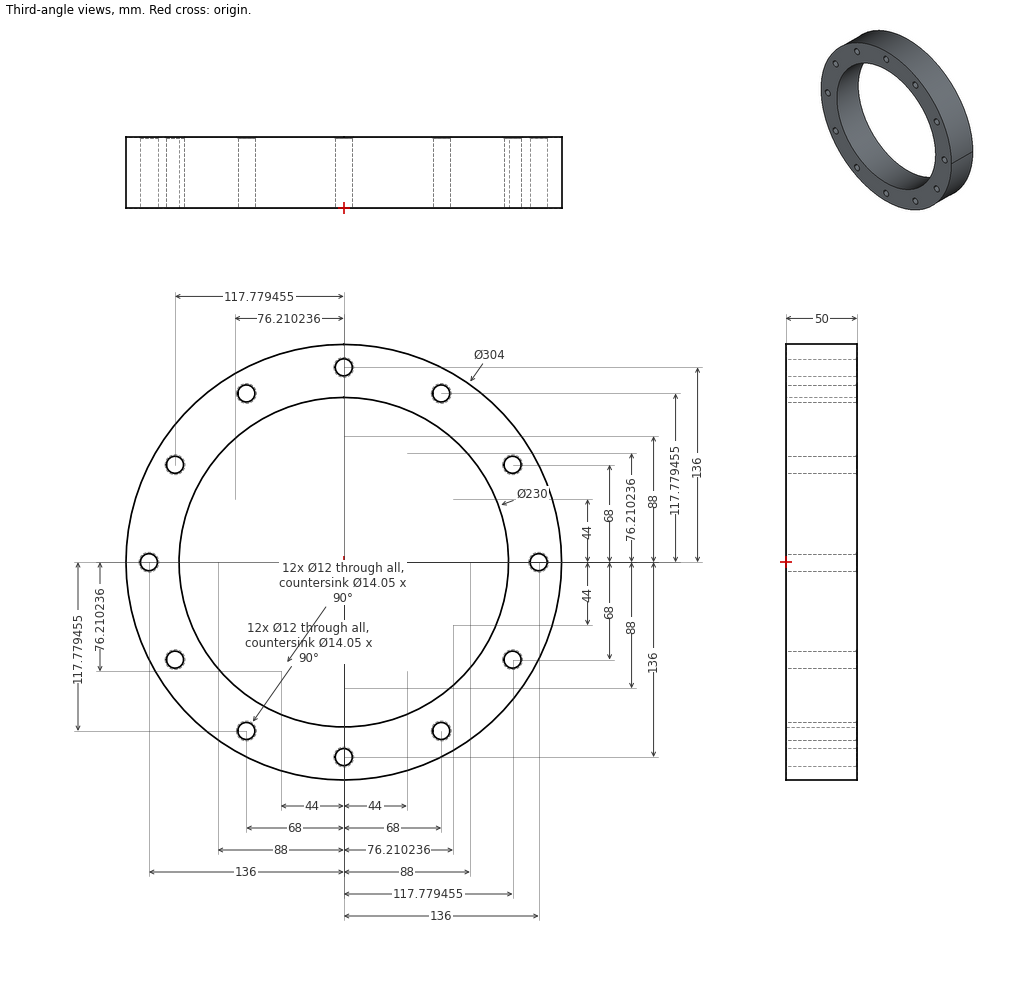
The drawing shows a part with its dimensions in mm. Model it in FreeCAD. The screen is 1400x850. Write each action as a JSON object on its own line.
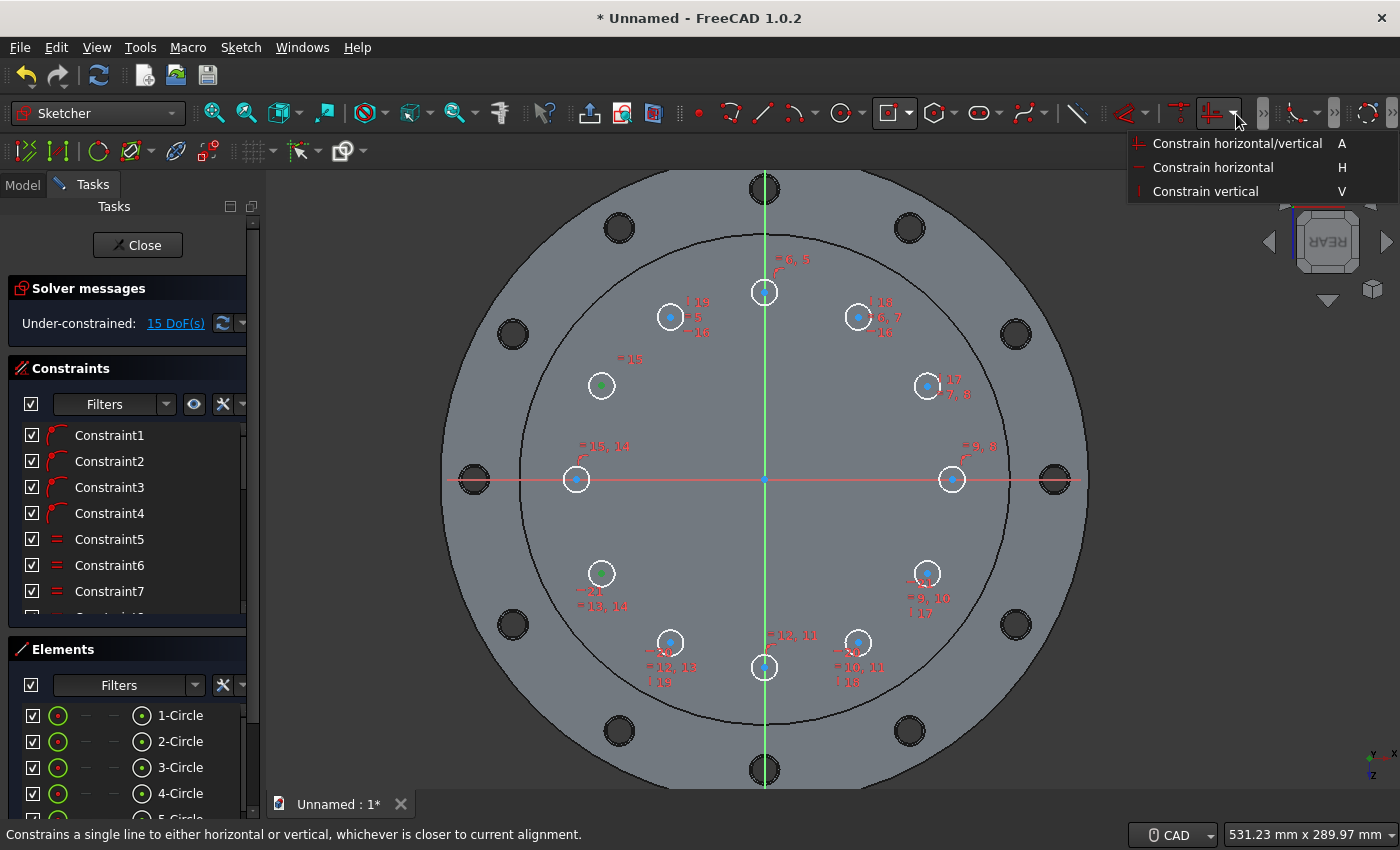
{"action": "left_click", "coordinate": [1263, 191]}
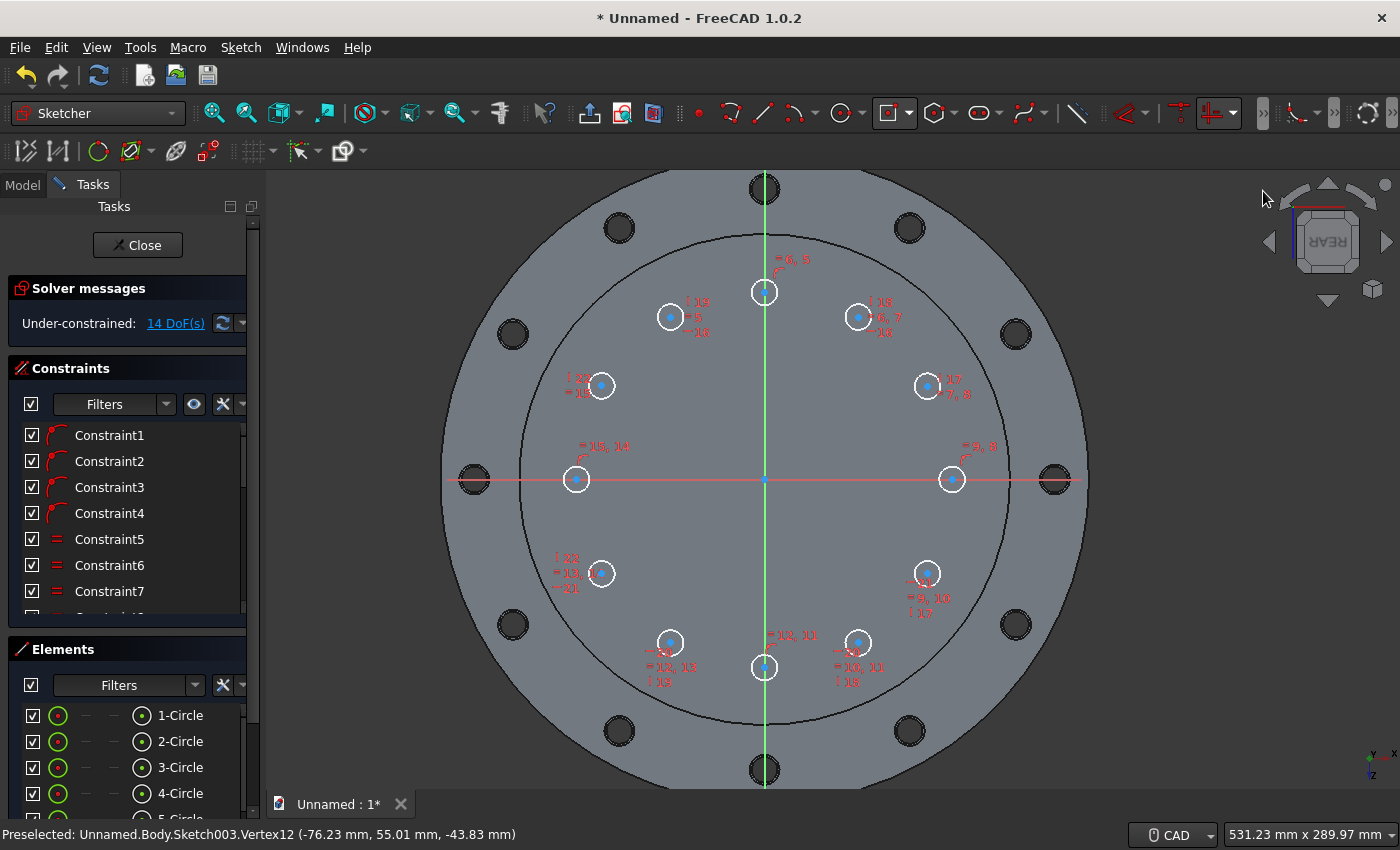
{"action": "left_click", "coordinate": [1124, 114]}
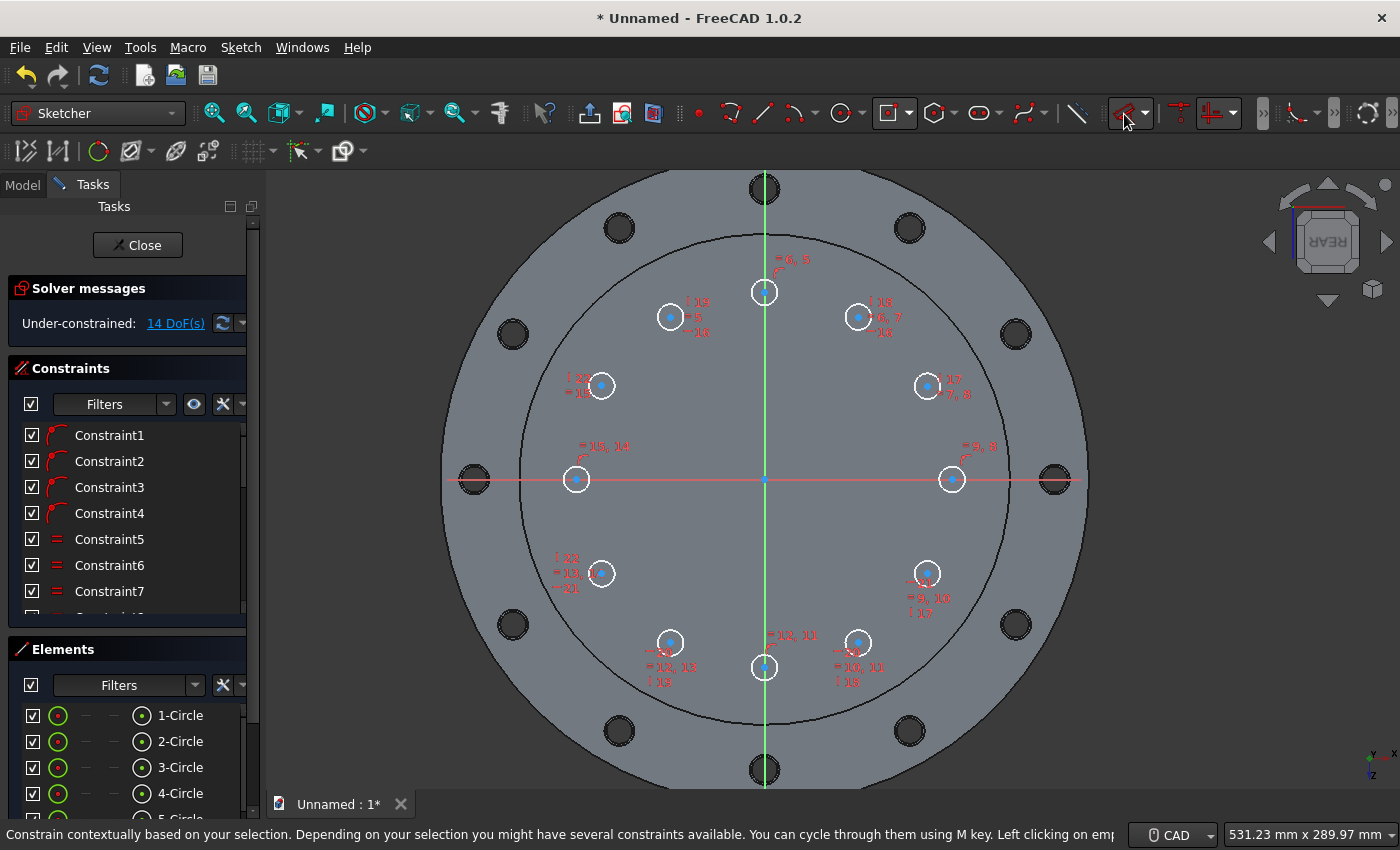
{"action": "scroll", "coordinate": [680, 308], "scroll_direction": "up", "scroll_amount": 3}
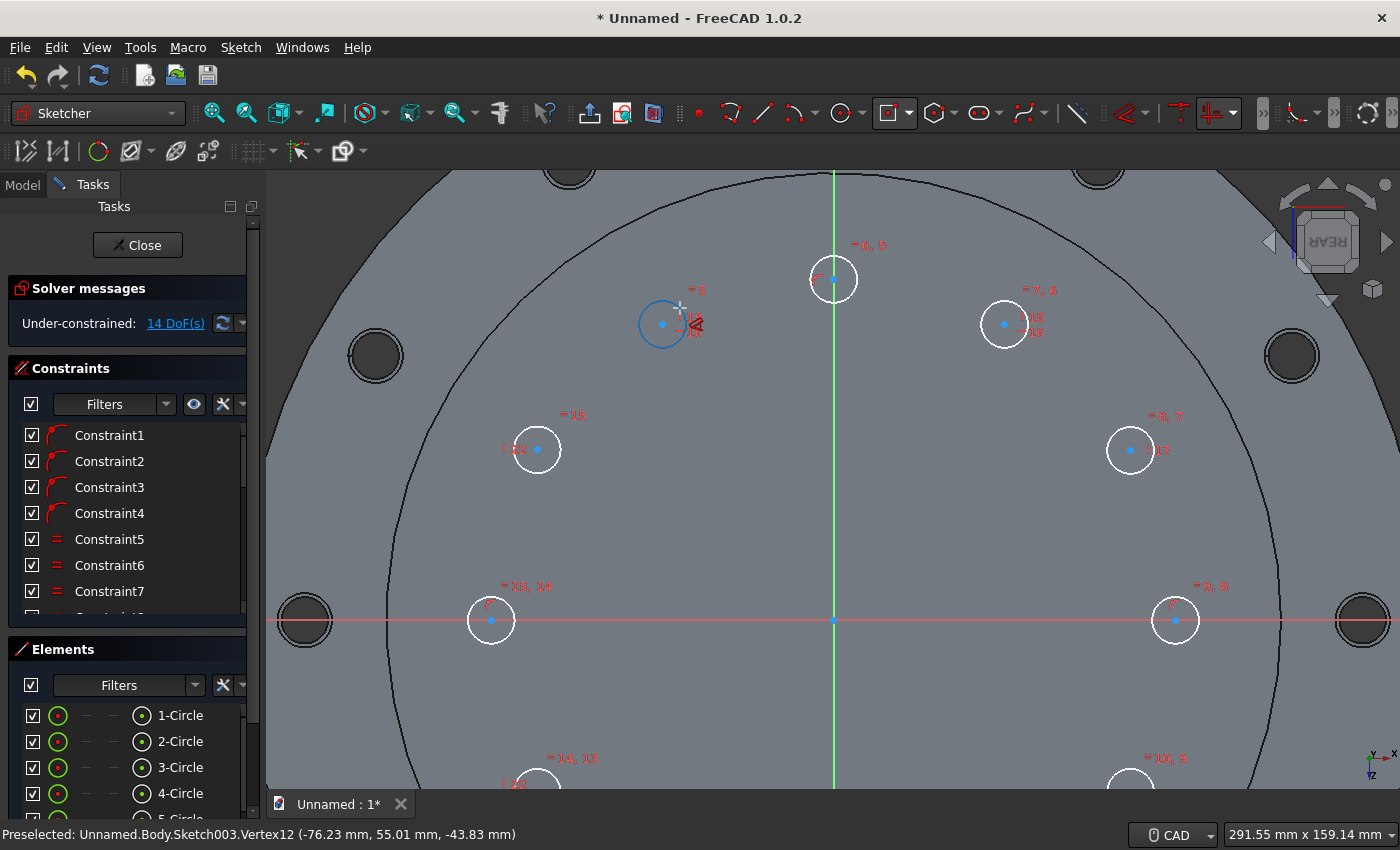
{"action": "left_click", "coordinate": [679, 308]}
{"action": "left_click", "coordinate": [702, 285]}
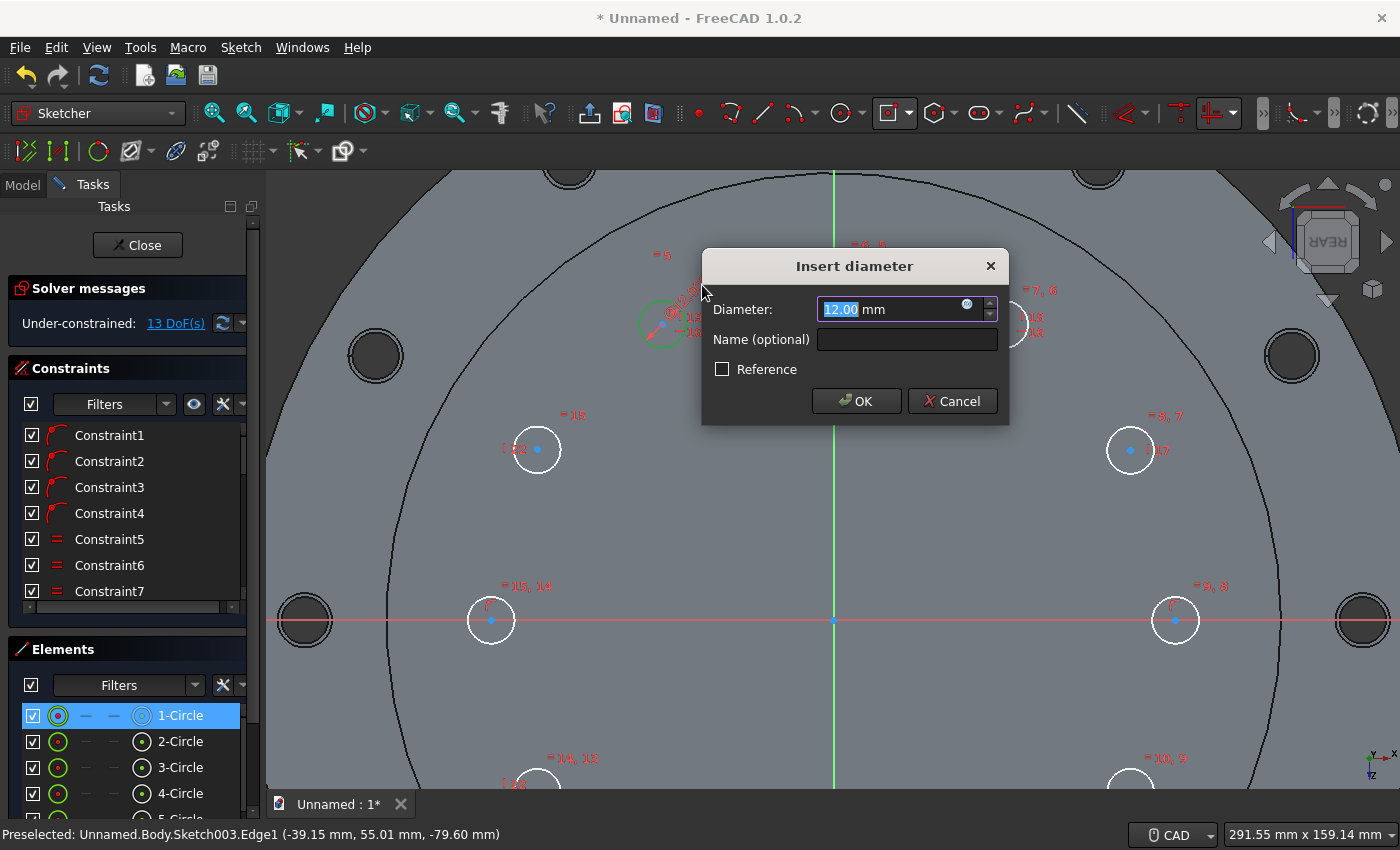
{"action": "type", "text": "12"}
{"action": "key", "text": "Return"}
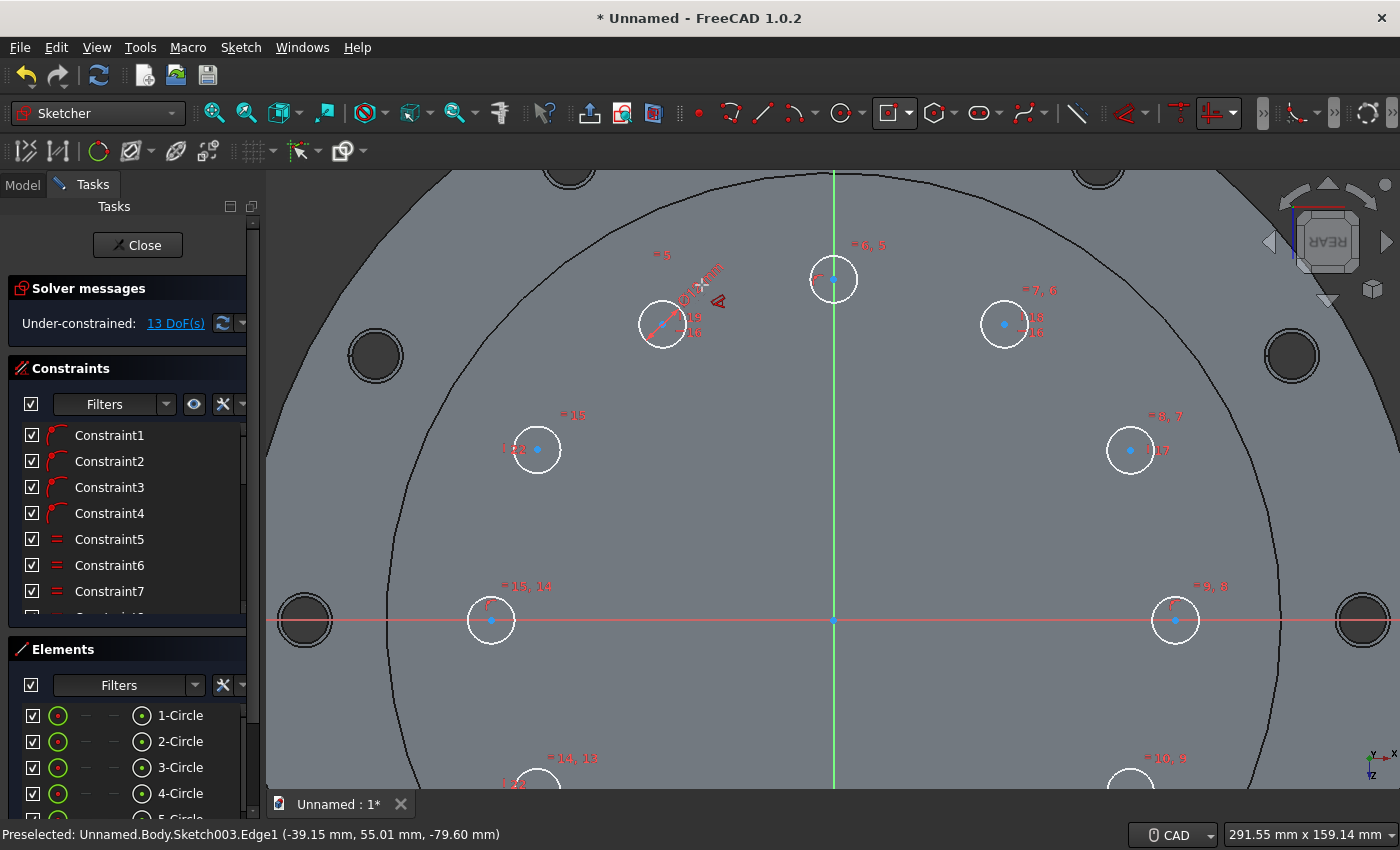
{"action": "left_click", "coordinate": [663, 324]}
{"action": "left_click", "coordinate": [788, 290]}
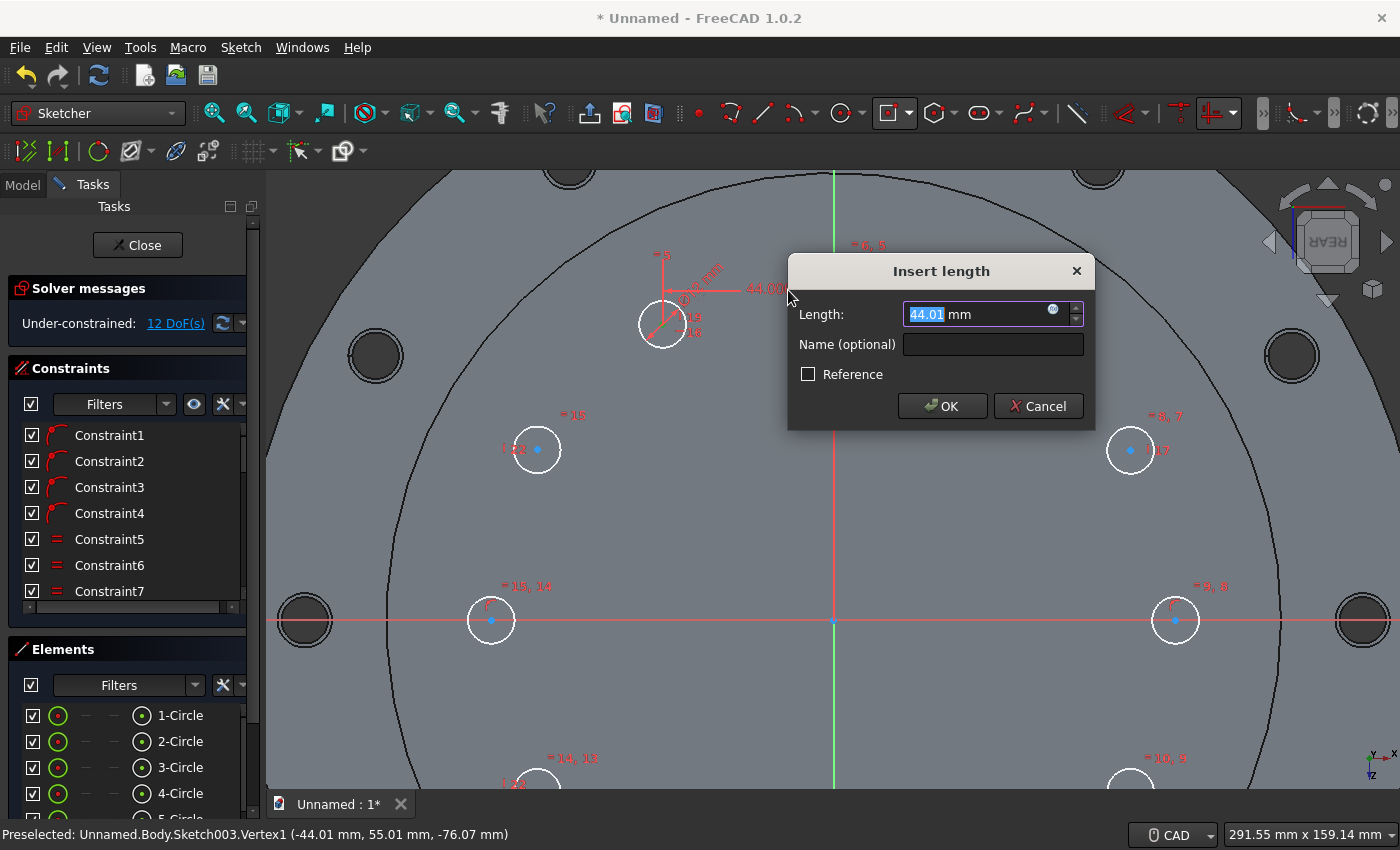
{"action": "type", "text": "44"}
{"action": "key", "text": "Return"}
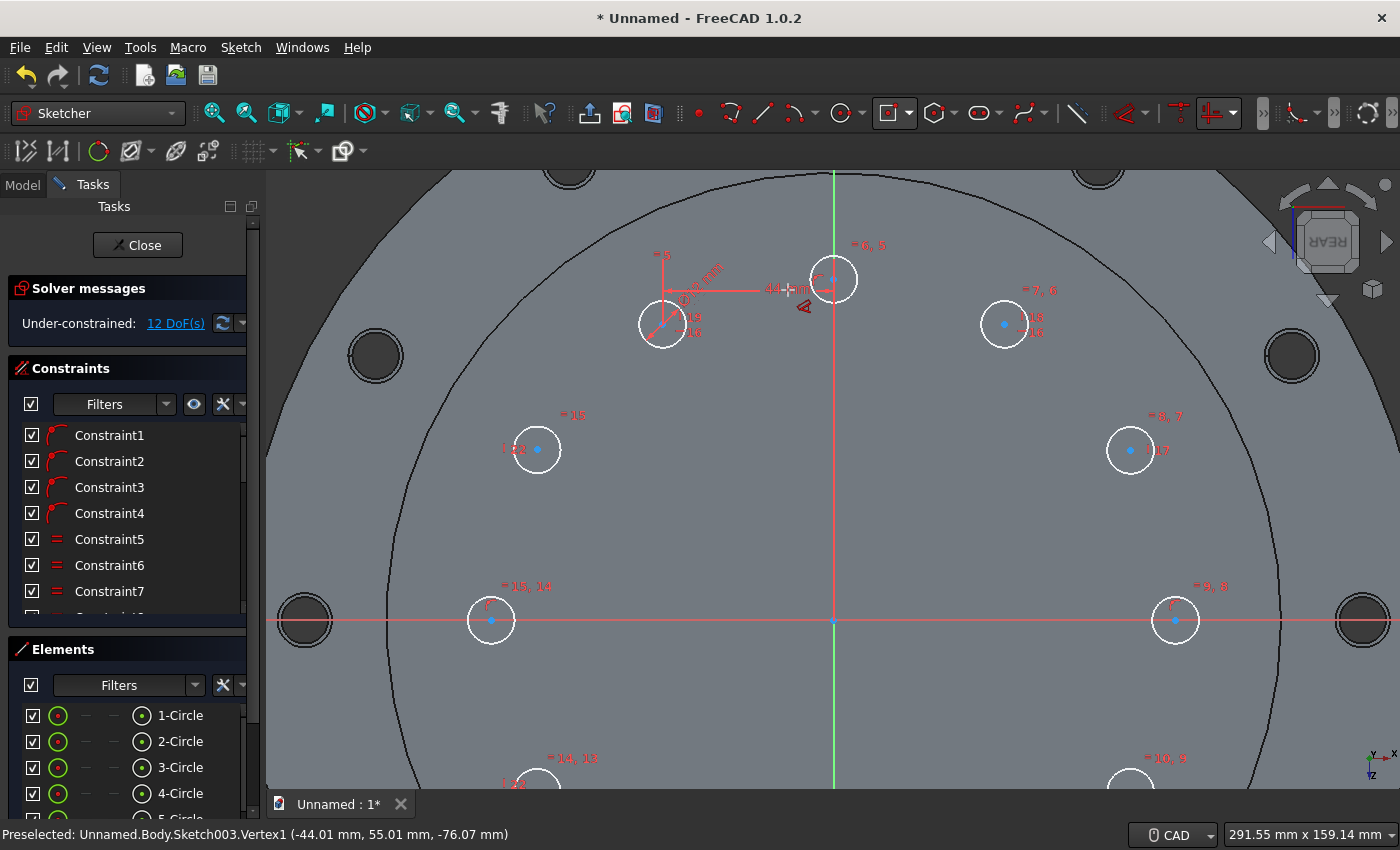
{"action": "left_click", "coordinate": [834, 279]}
{"action": "left_click", "coordinate": [868, 450]}